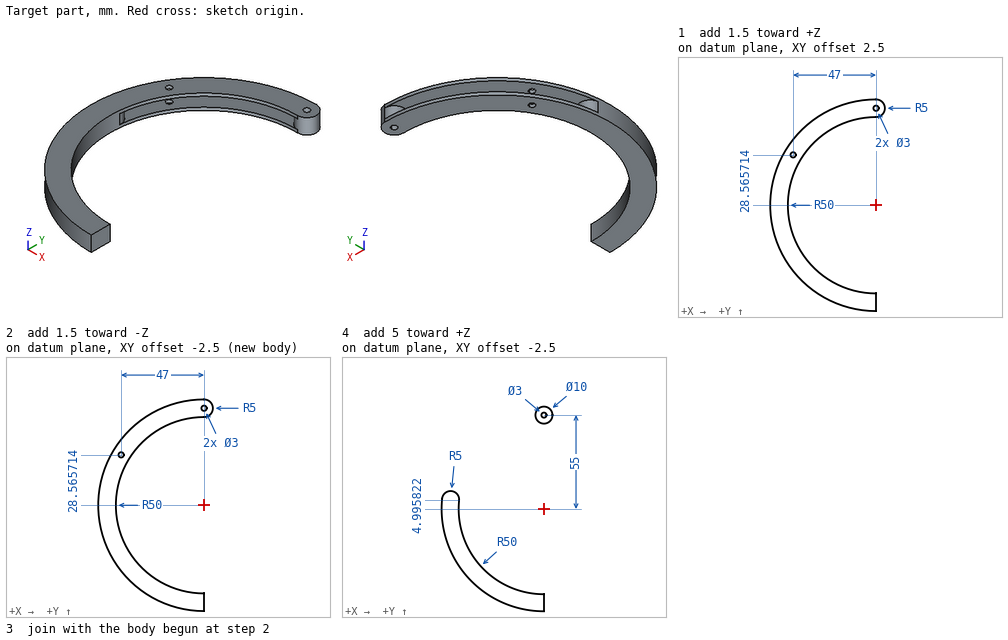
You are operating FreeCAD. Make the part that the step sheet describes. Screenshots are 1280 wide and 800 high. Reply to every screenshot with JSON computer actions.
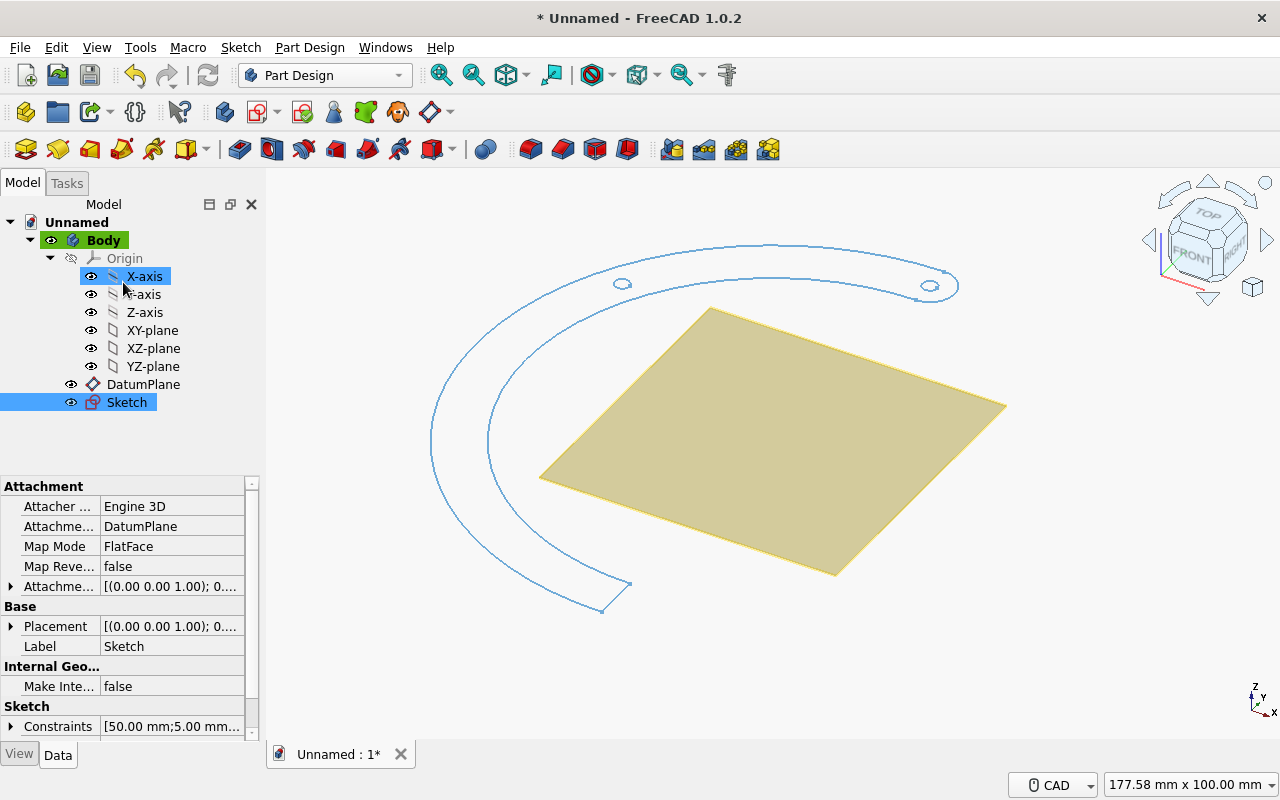
{"action": "left_click", "coordinate": [26, 150]}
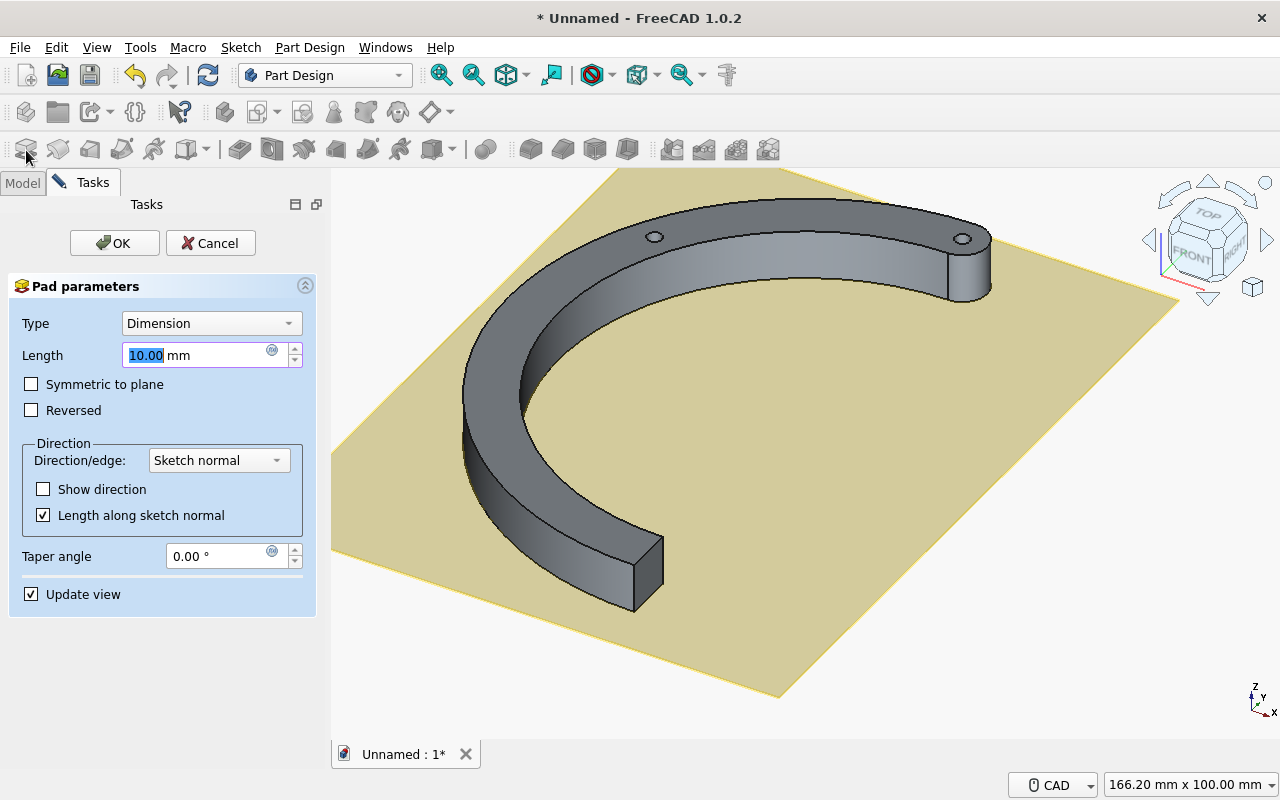
{"action": "type", "text": "1.5"}
{"action": "key", "text": "Tab"}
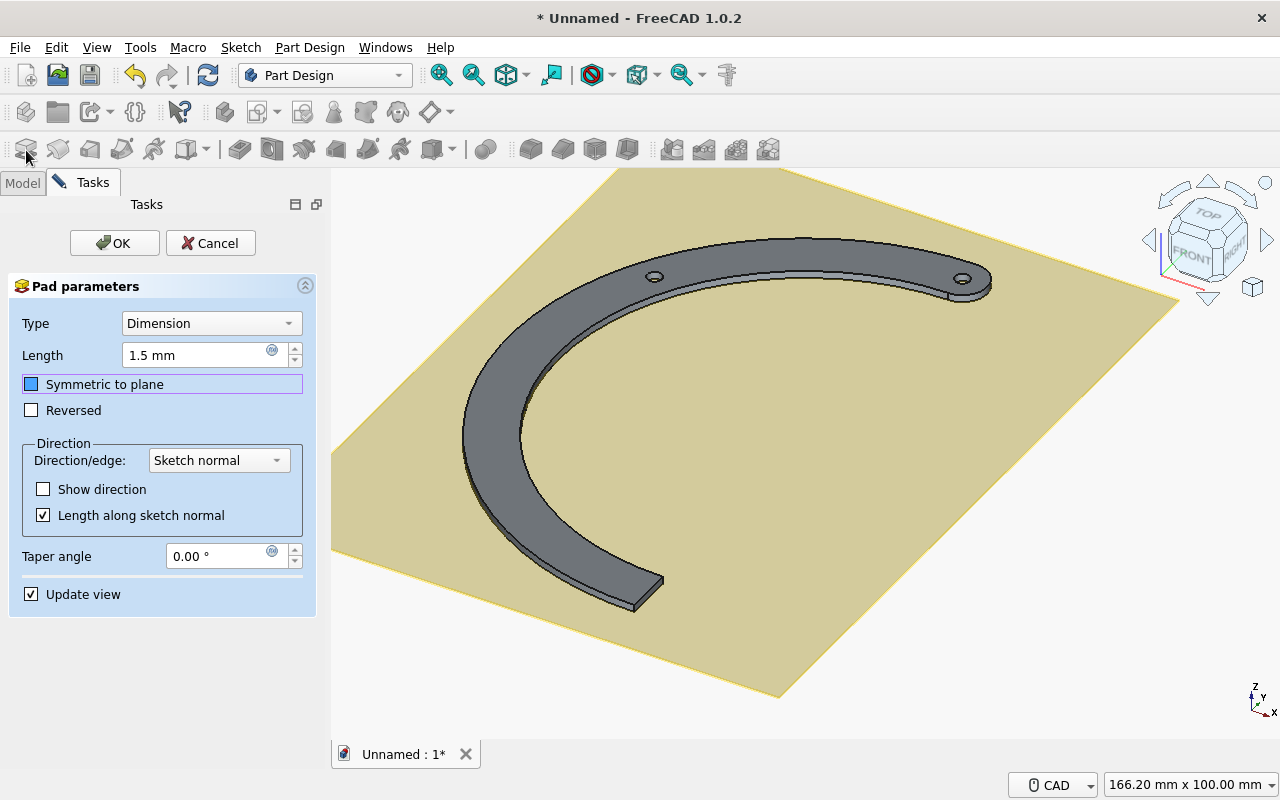
{"action": "left_click", "coordinate": [115, 243]}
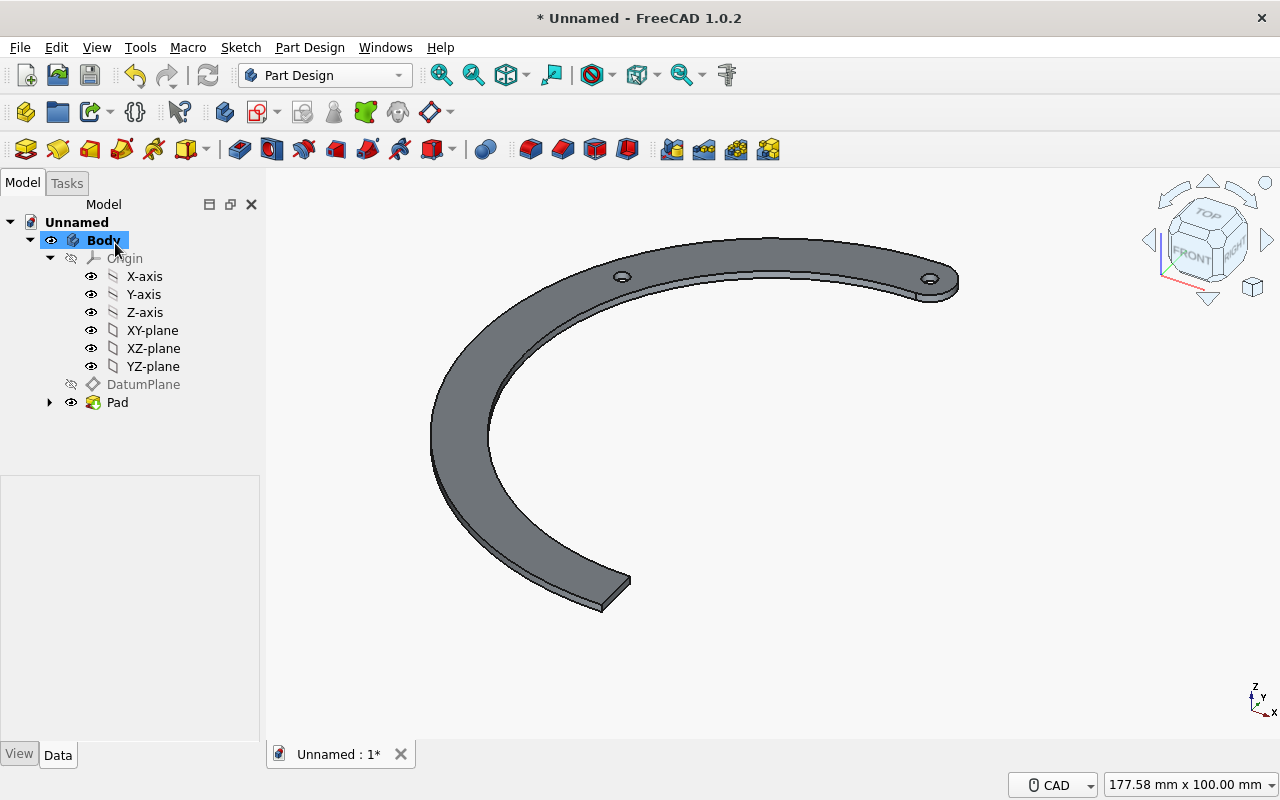
{"action": "left_click", "coordinate": [442, 76]}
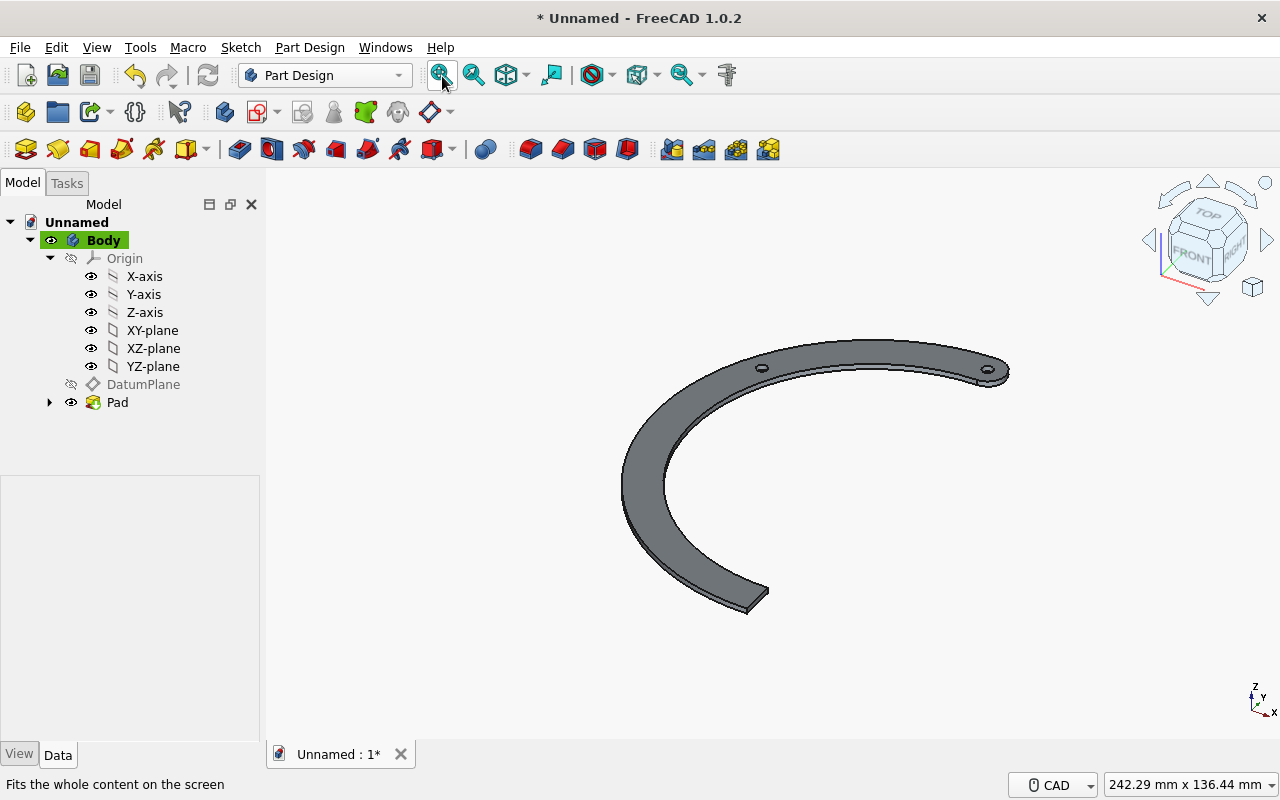
{"action": "left_click", "coordinate": [226, 112]}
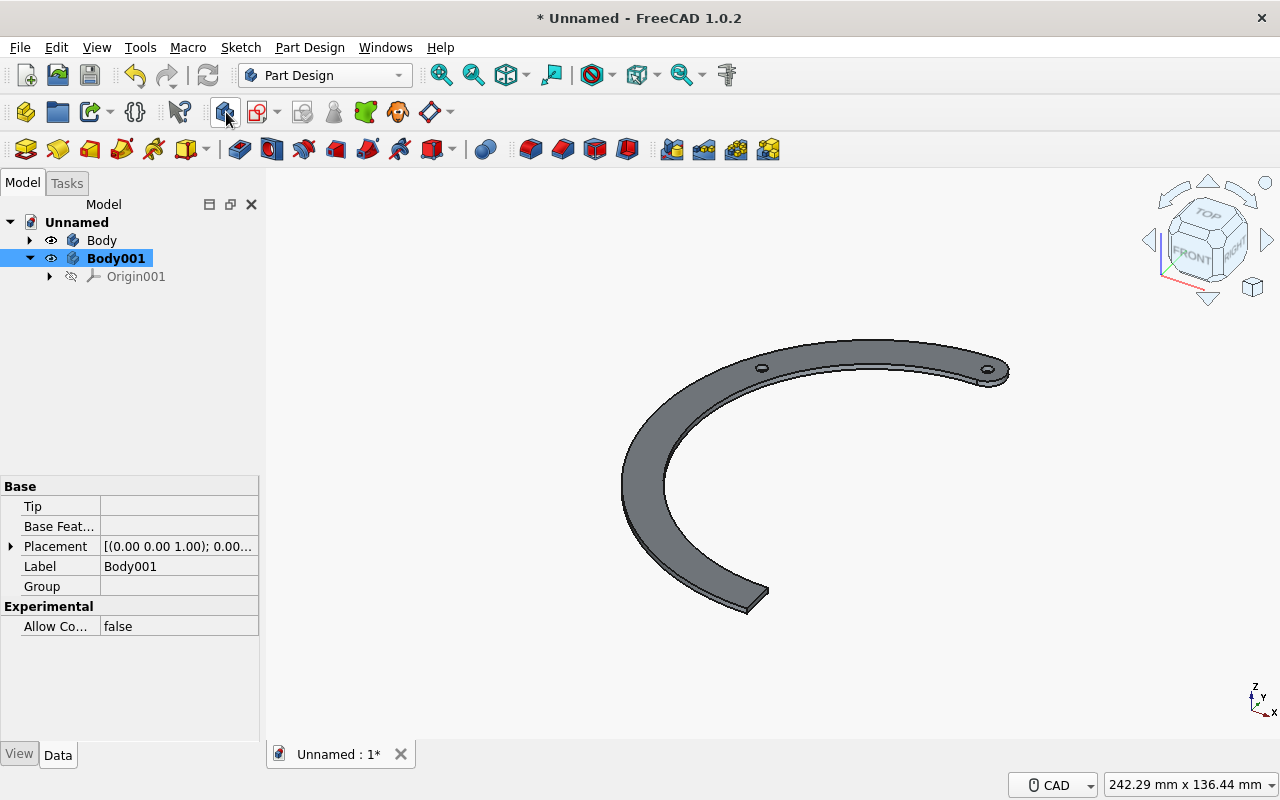
{"action": "left_click", "coordinate": [50, 276]}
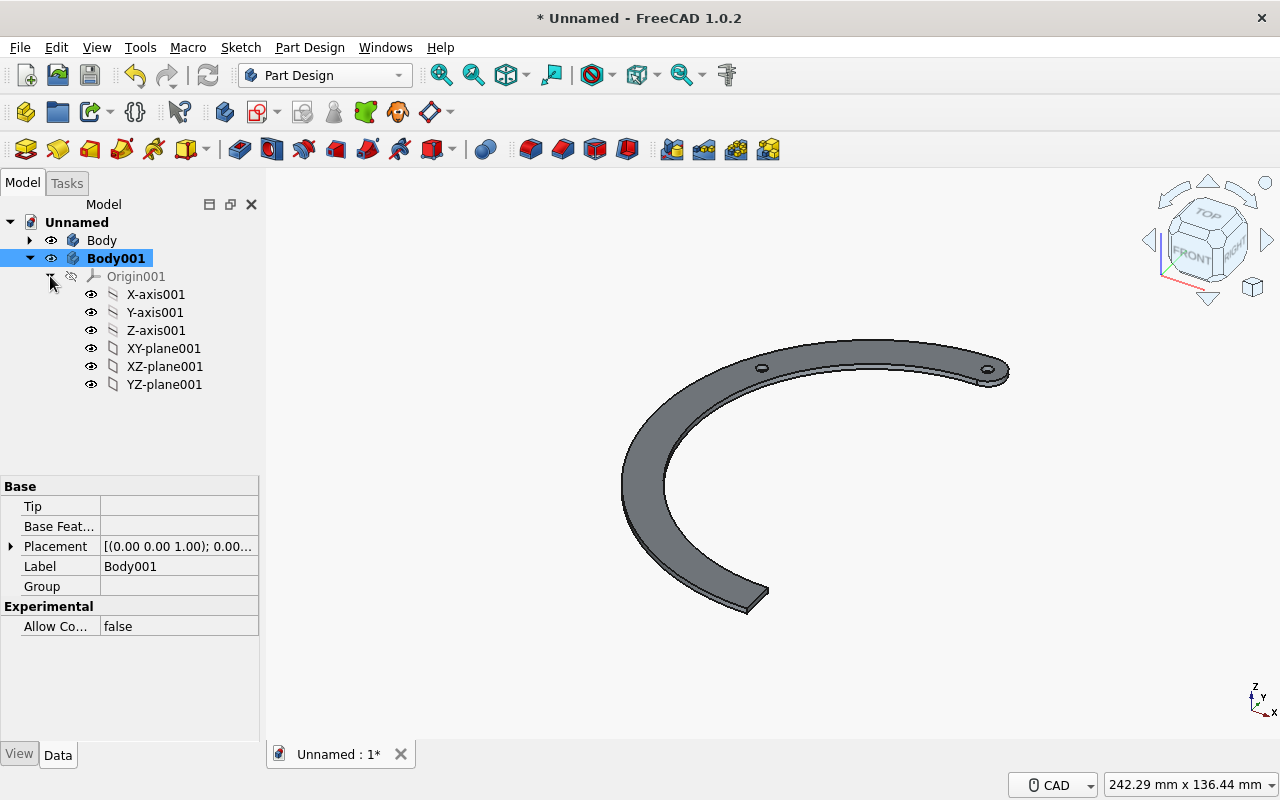
{"action": "left_click", "coordinate": [136, 348]}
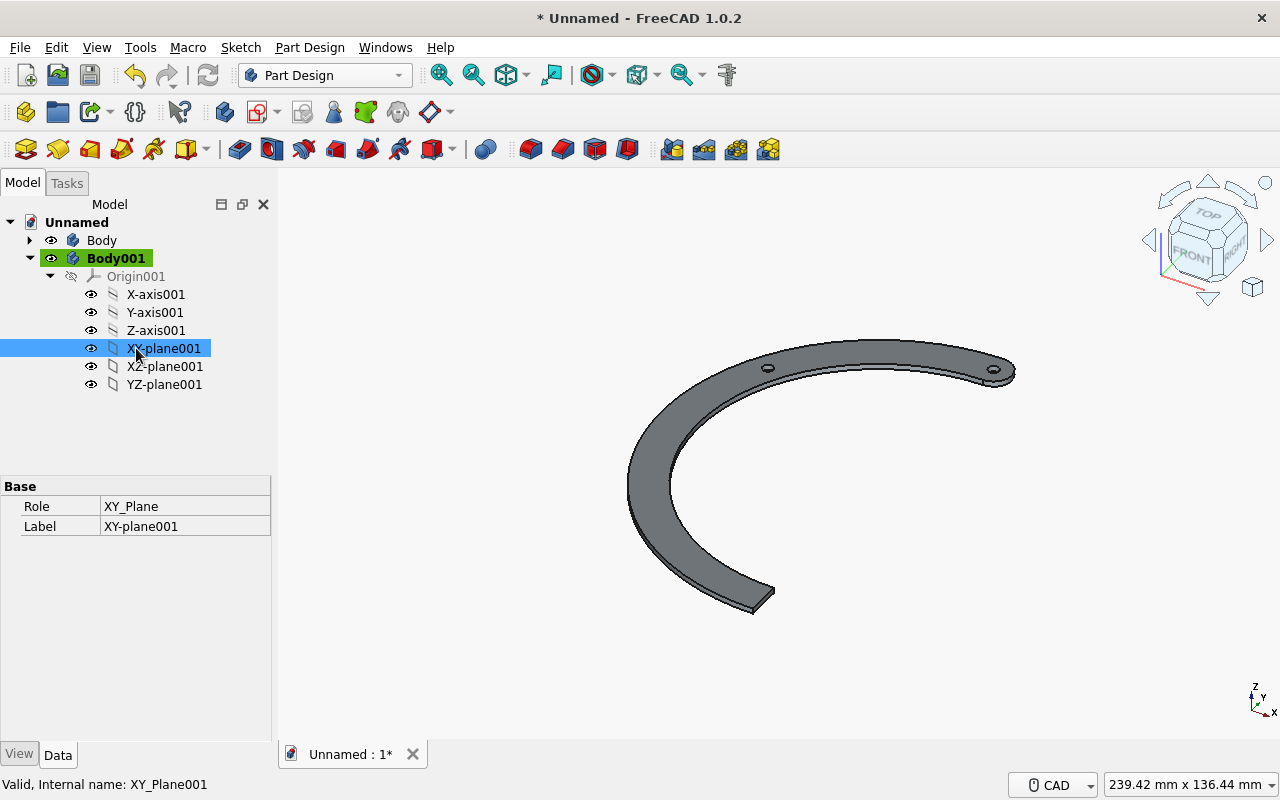
{"action": "left_click", "coordinate": [430, 112]}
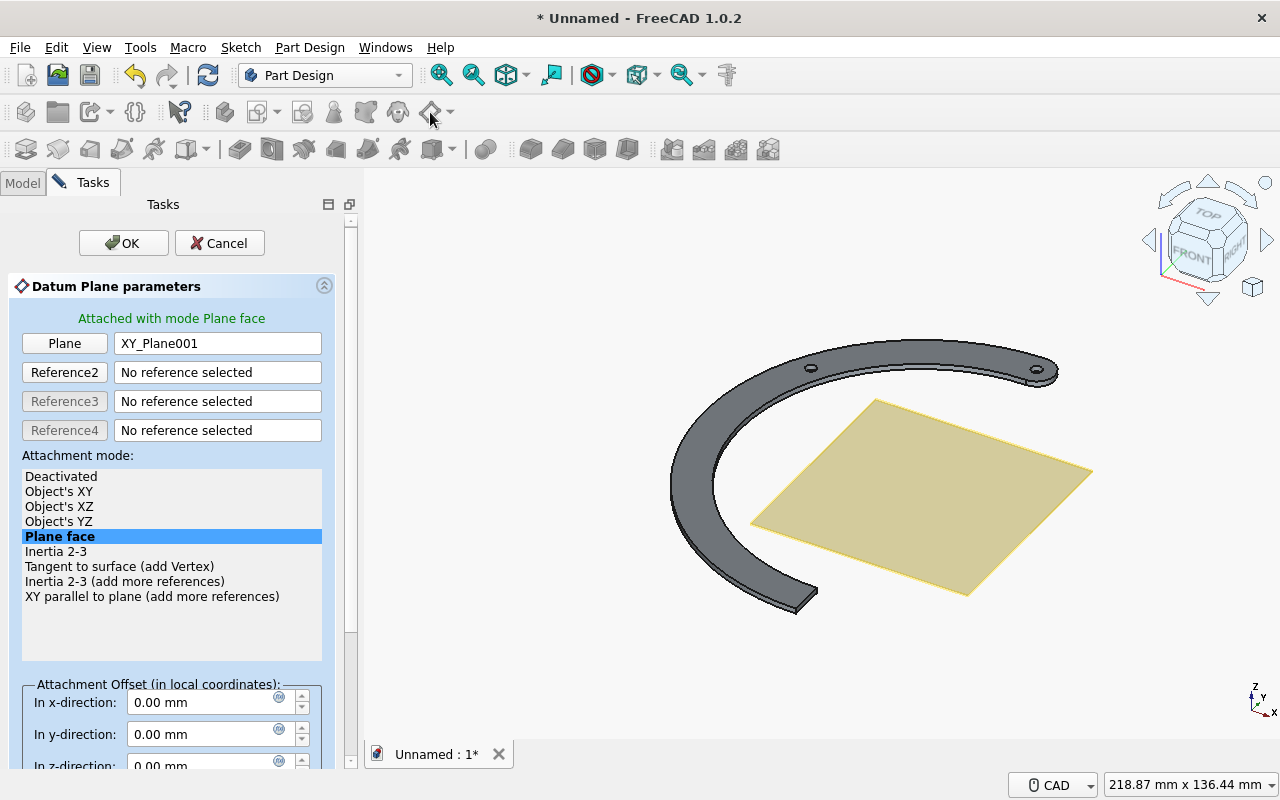
{"action": "scroll", "coordinate": [351, 491], "scroll_direction": "down", "scroll_amount": 2}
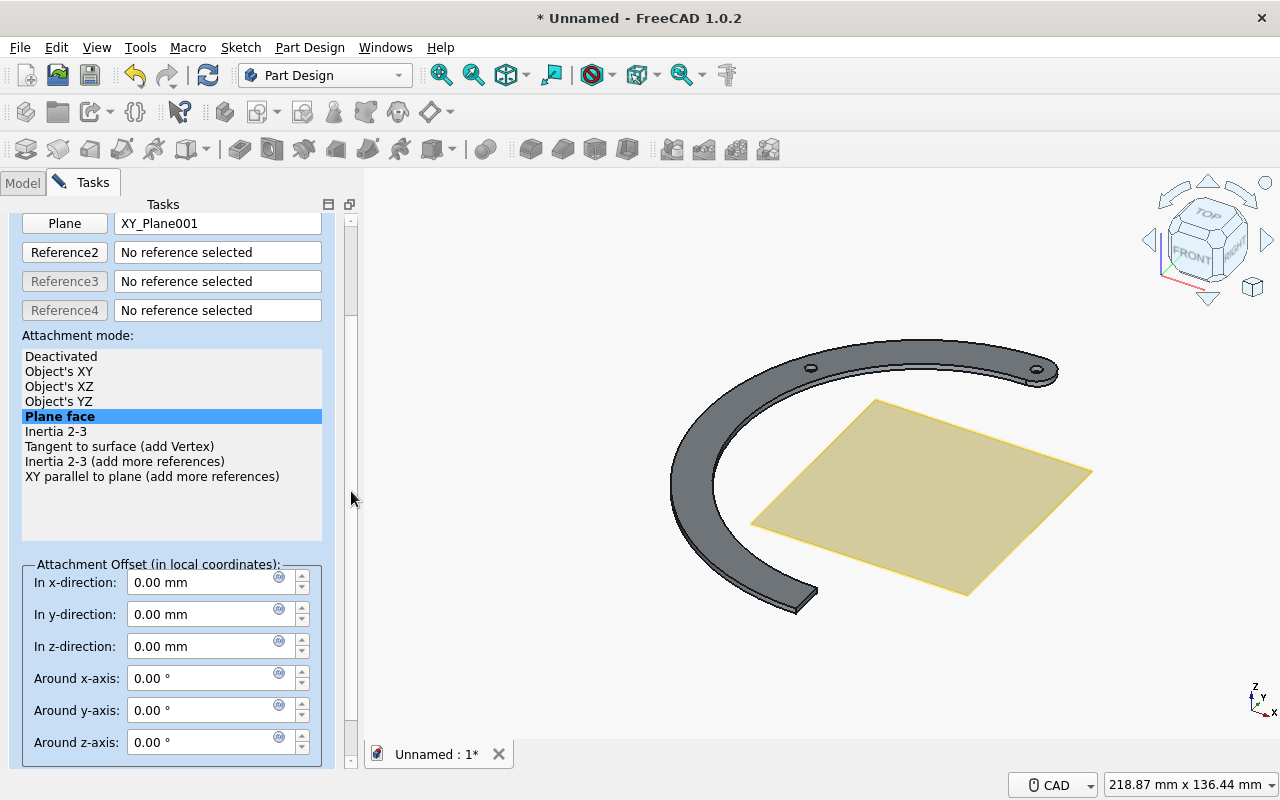
{"action": "triple_click", "coordinate": [210, 646]}